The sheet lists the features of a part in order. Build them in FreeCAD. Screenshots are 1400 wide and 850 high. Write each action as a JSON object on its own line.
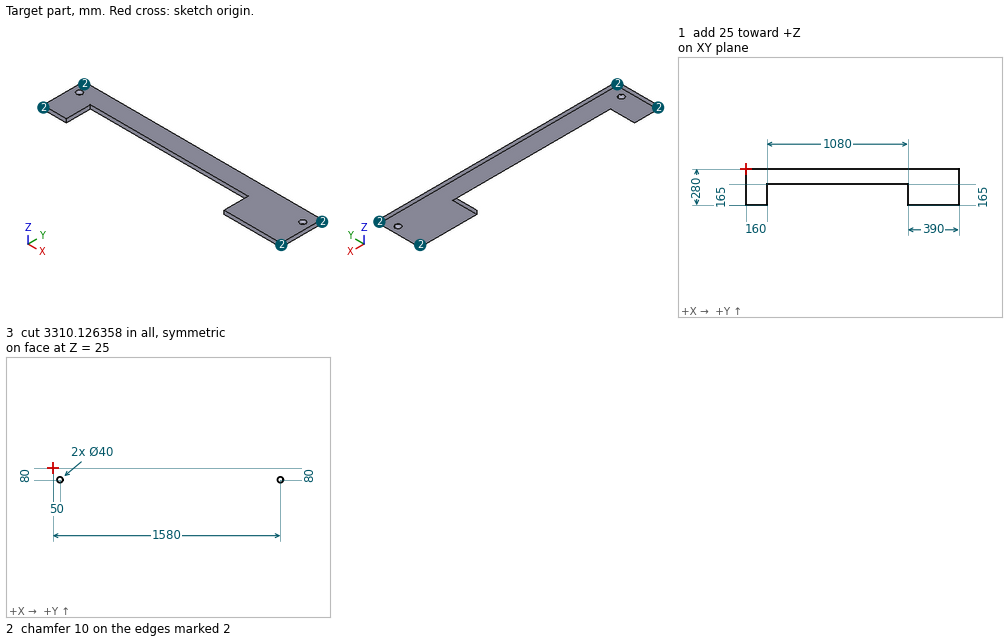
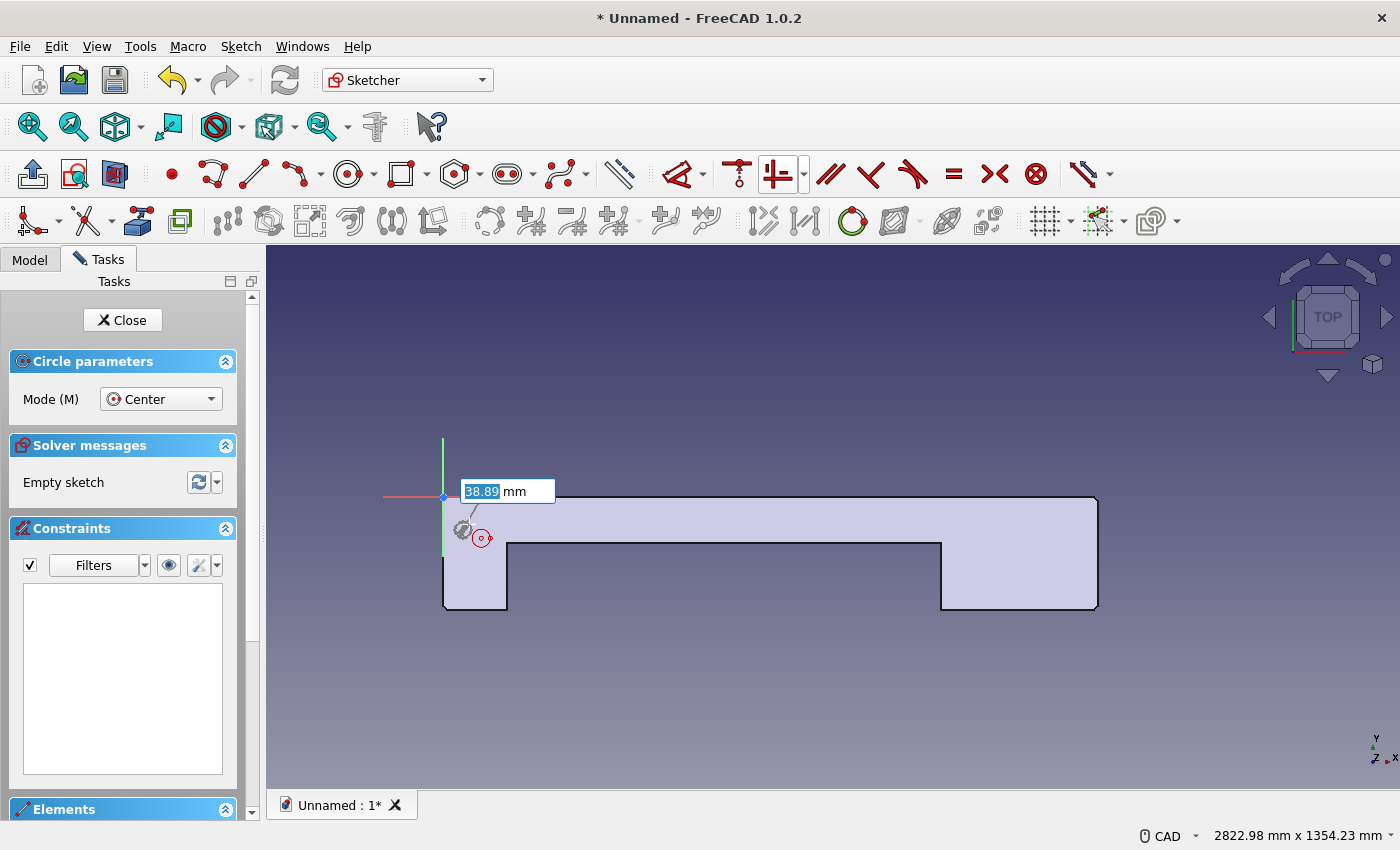
{"action": "type", "text": "40"}
{"action": "key", "text": "Return"}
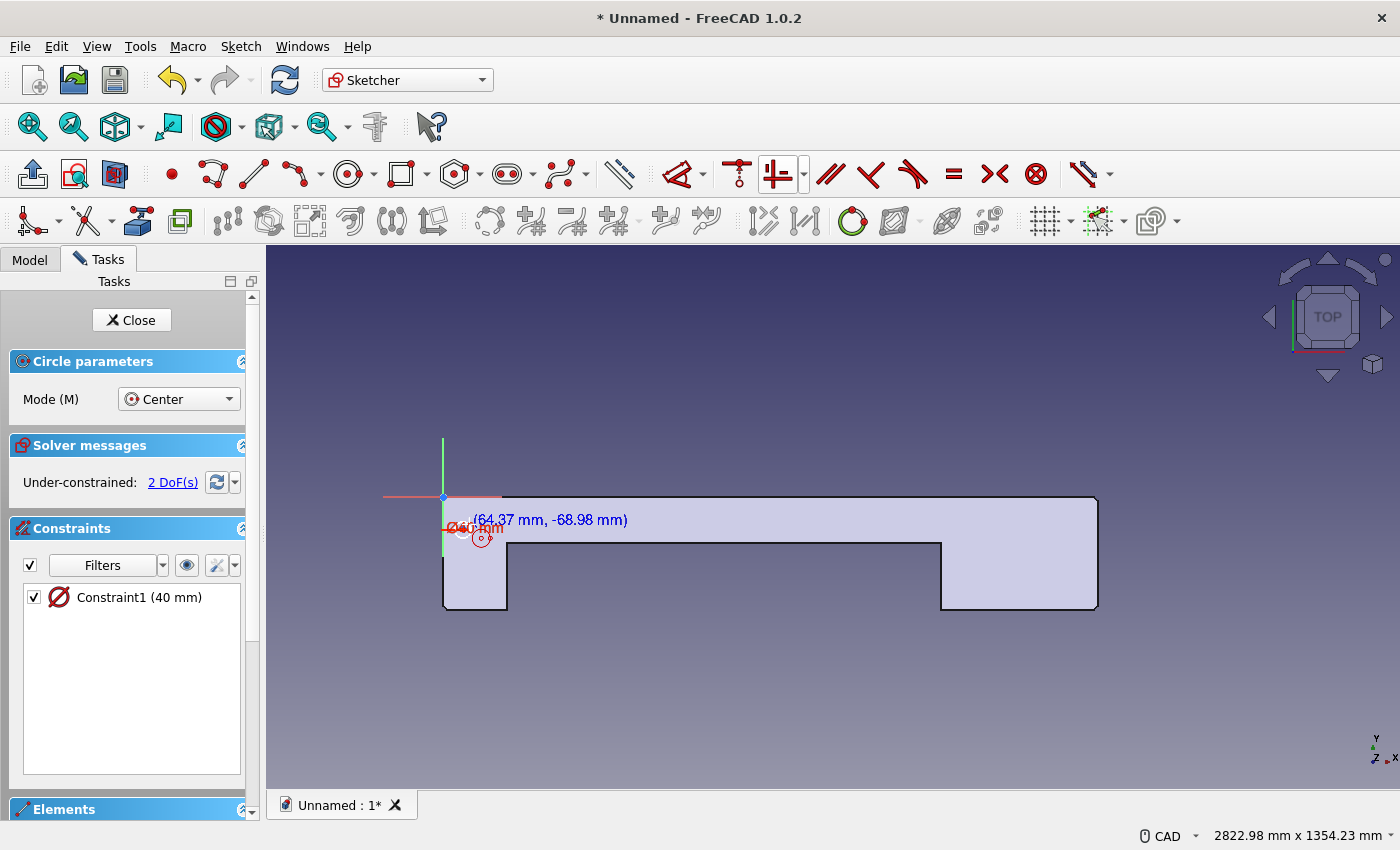
{"action": "scroll", "coordinate": [1078, 529], "scroll_direction": "up", "scroll_amount": 6}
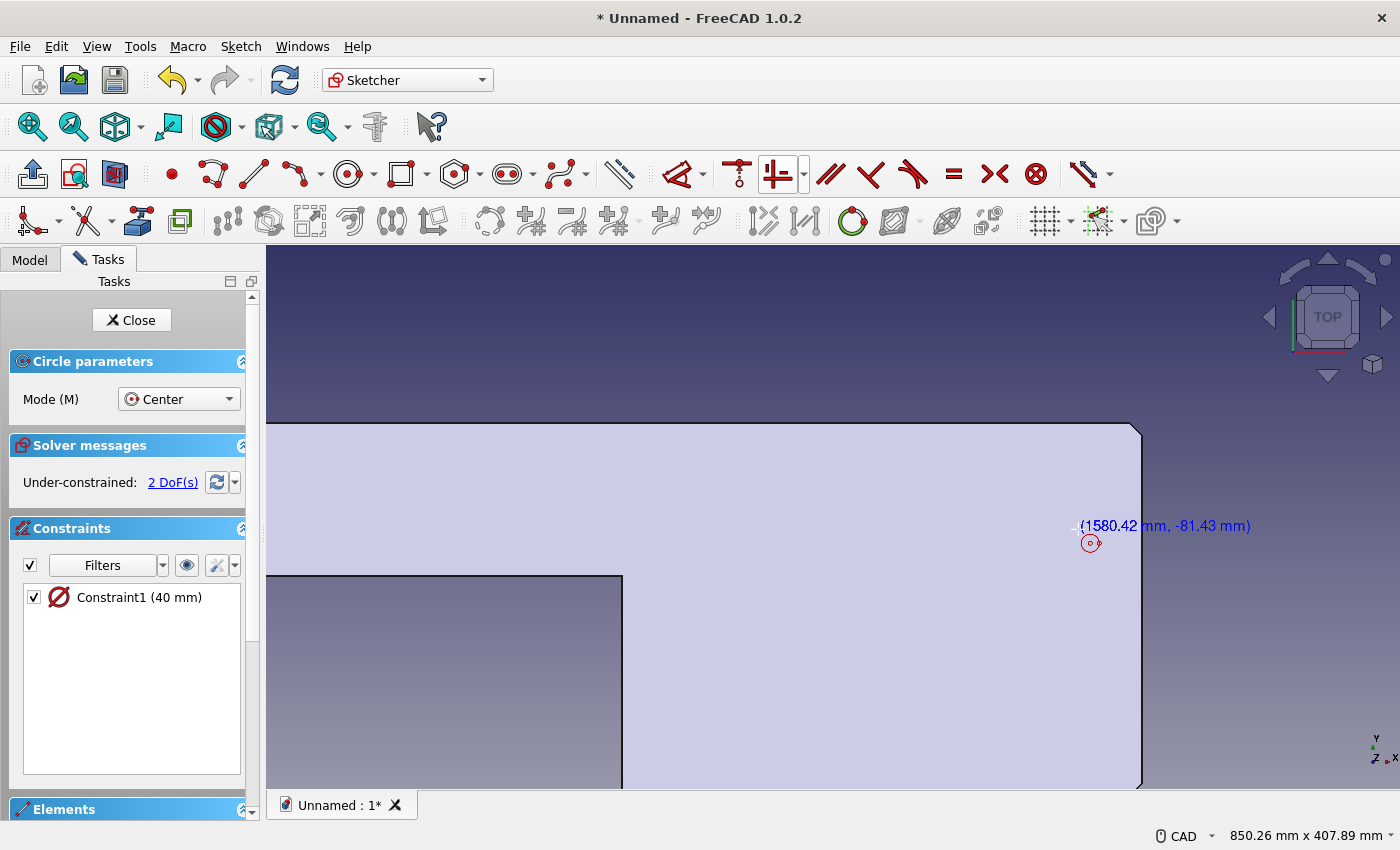
{"action": "scroll", "coordinate": [1079, 529], "scroll_direction": "down", "scroll_amount": 6}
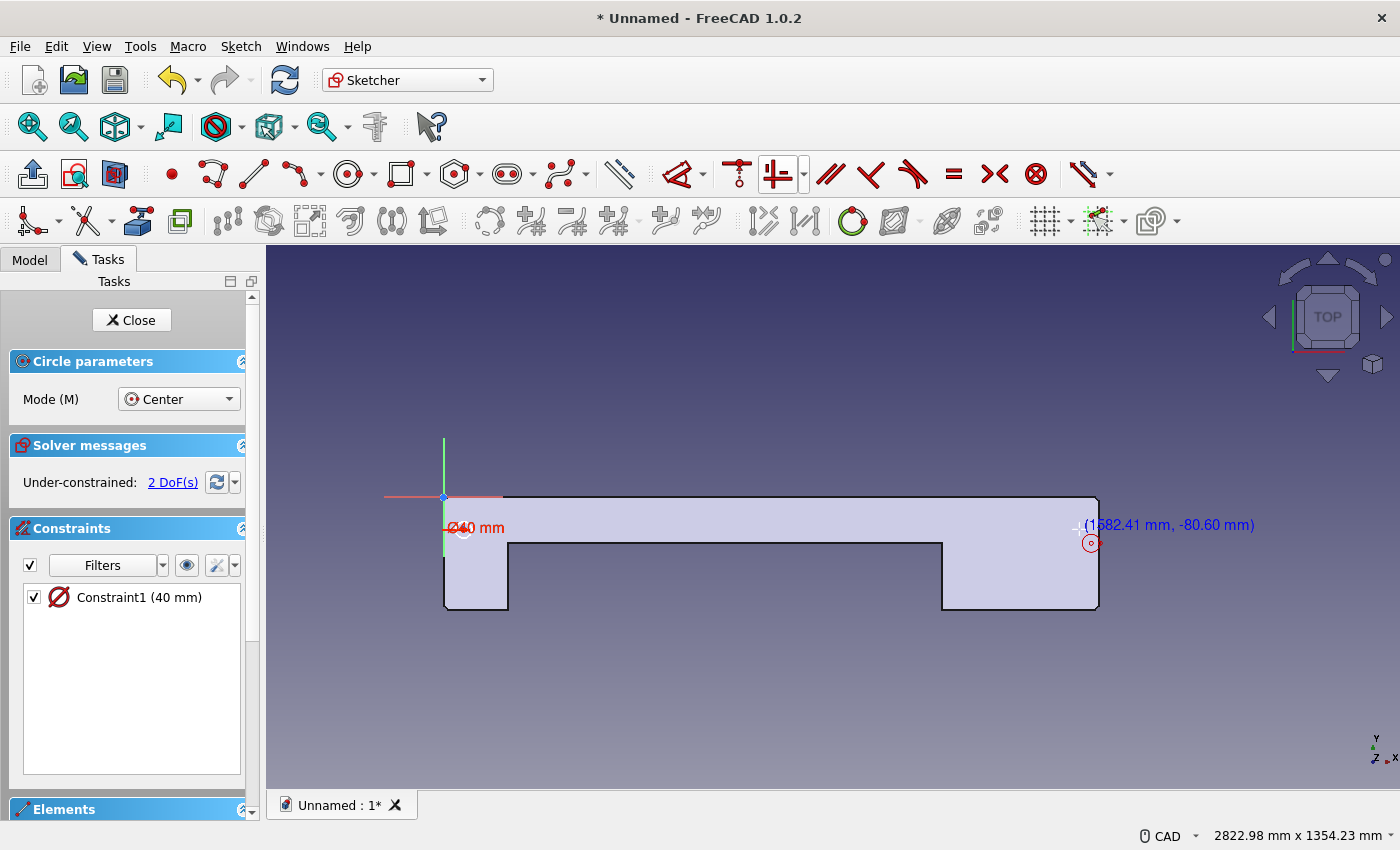
{"action": "left_click", "coordinate": [1079, 529]}
{"action": "mouse_move", "coordinate": [1084, 524]}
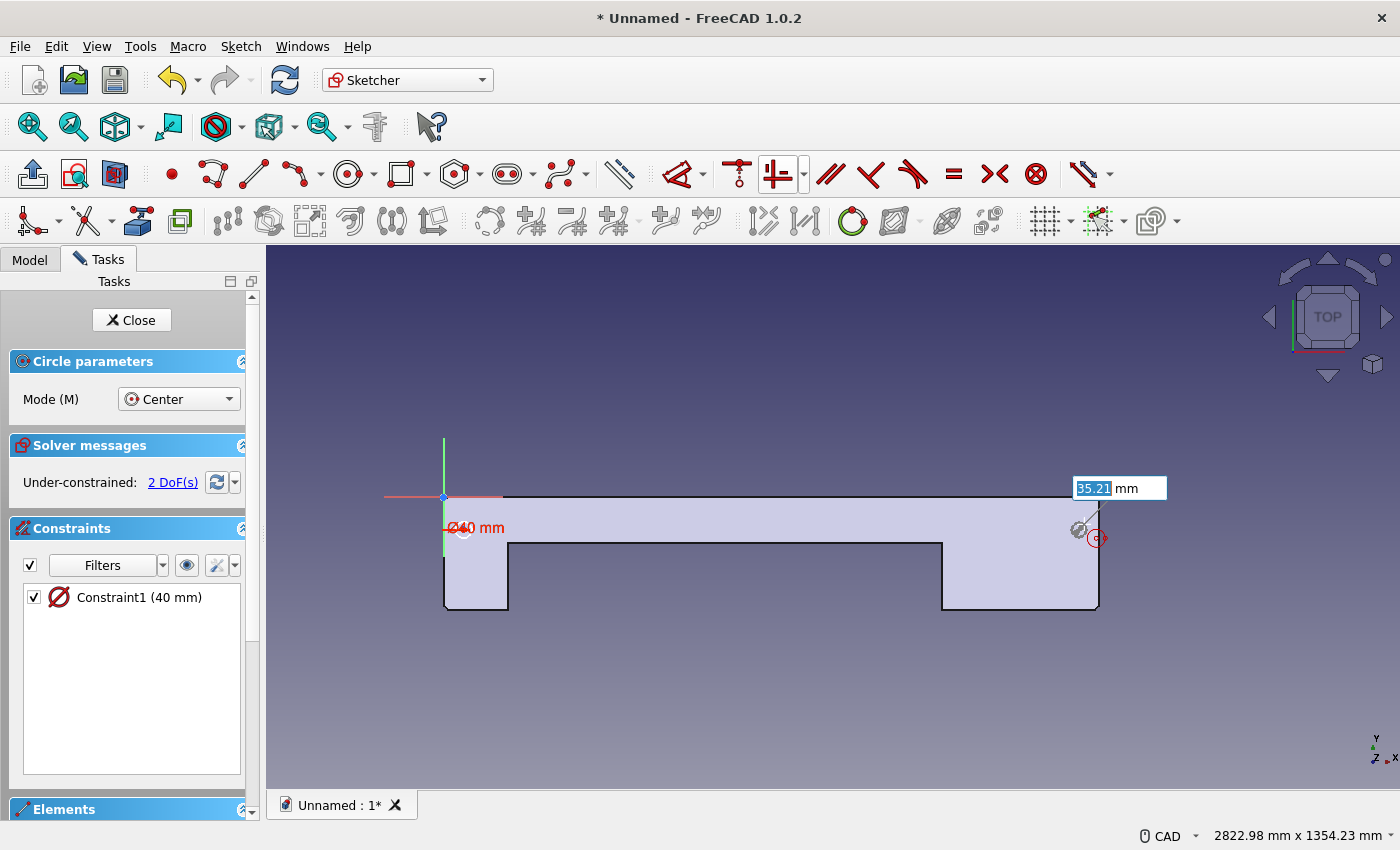
{"action": "type", "text": "40"}
{"action": "key", "text": "Return"}
{"action": "key", "text": "Escape"}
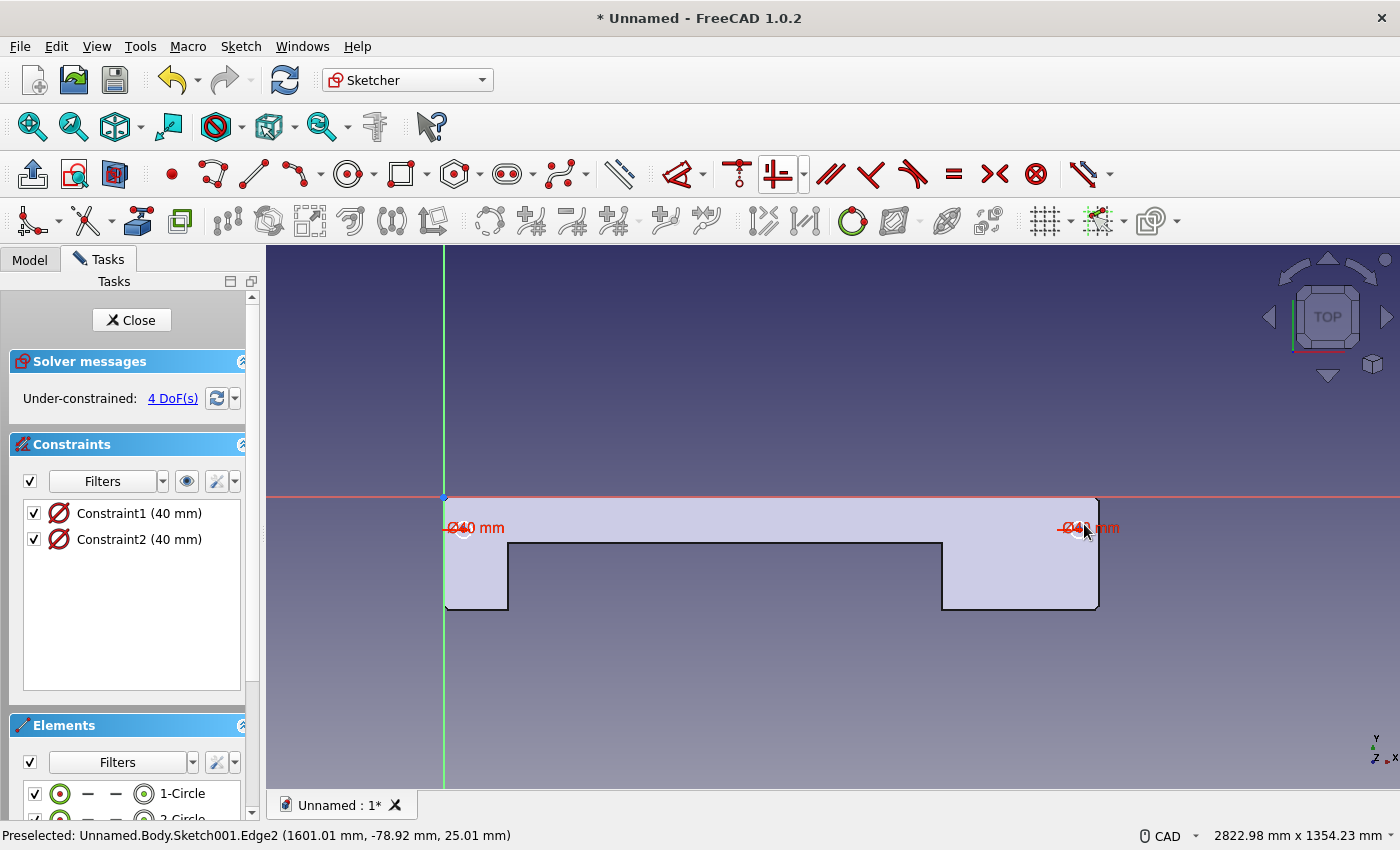
{"action": "left_click", "coordinate": [676, 174]}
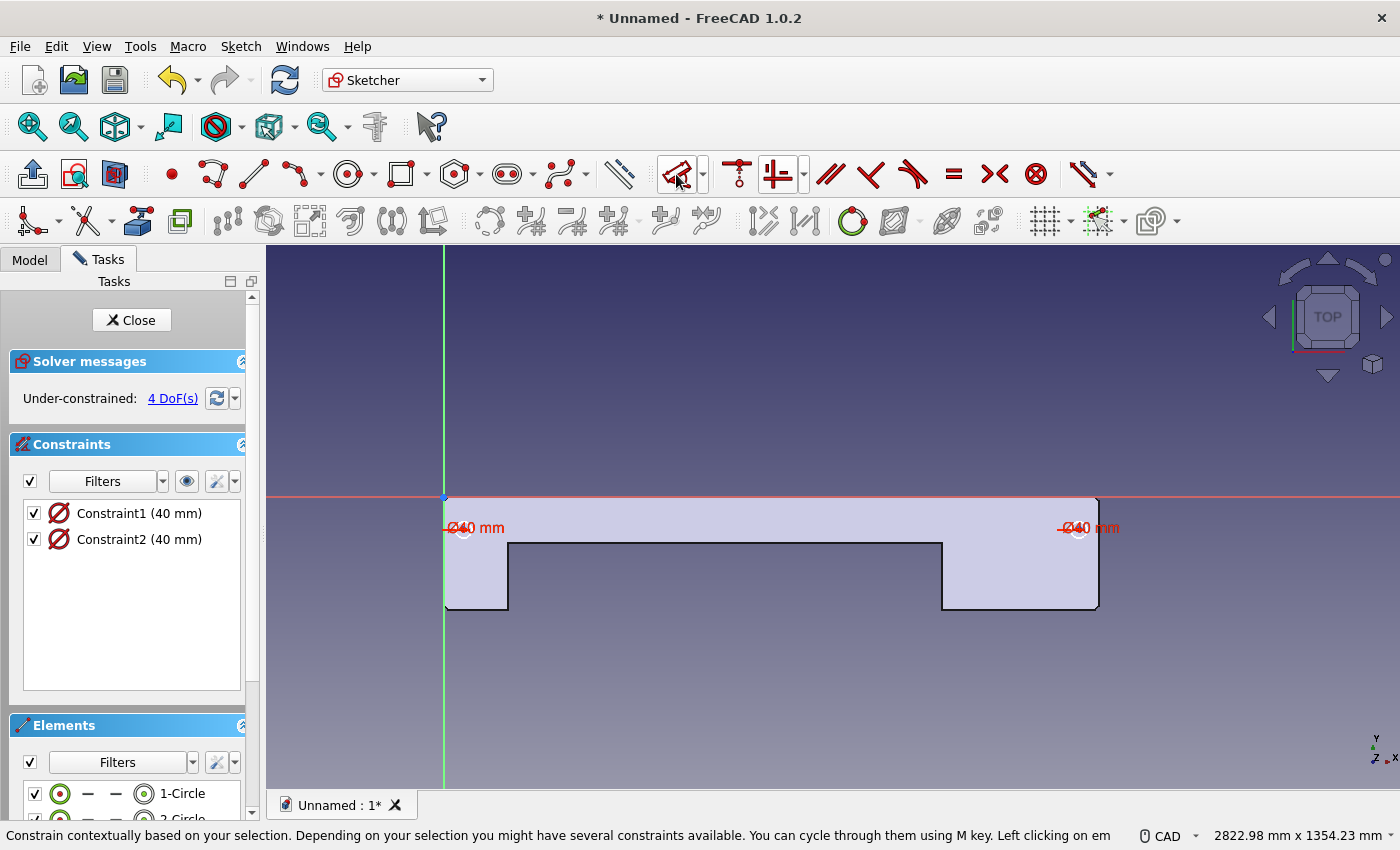
{"action": "scroll", "coordinate": [464, 530], "scroll_direction": "up", "scroll_amount": 4}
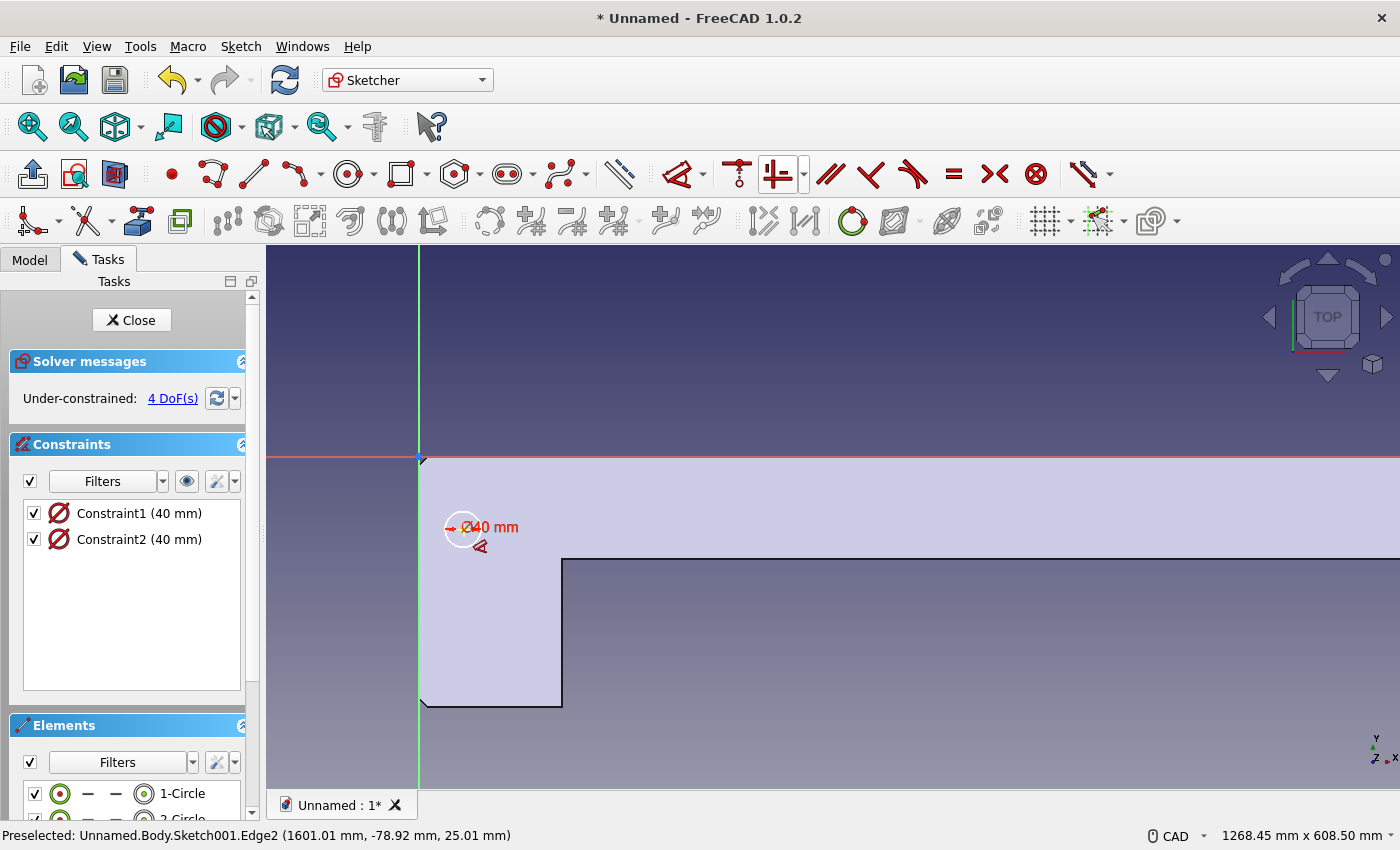
{"action": "left_click", "coordinate": [463, 529]}
{"action": "left_click", "coordinate": [441, 423]}